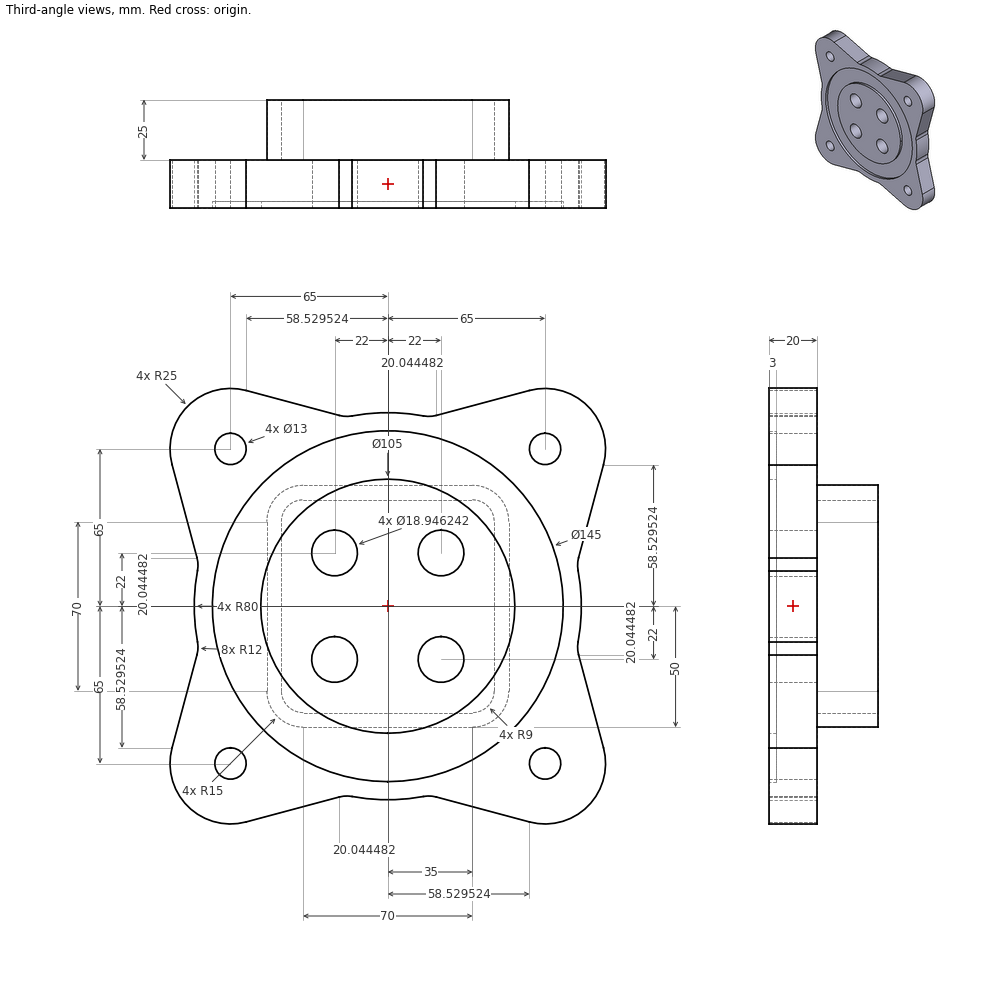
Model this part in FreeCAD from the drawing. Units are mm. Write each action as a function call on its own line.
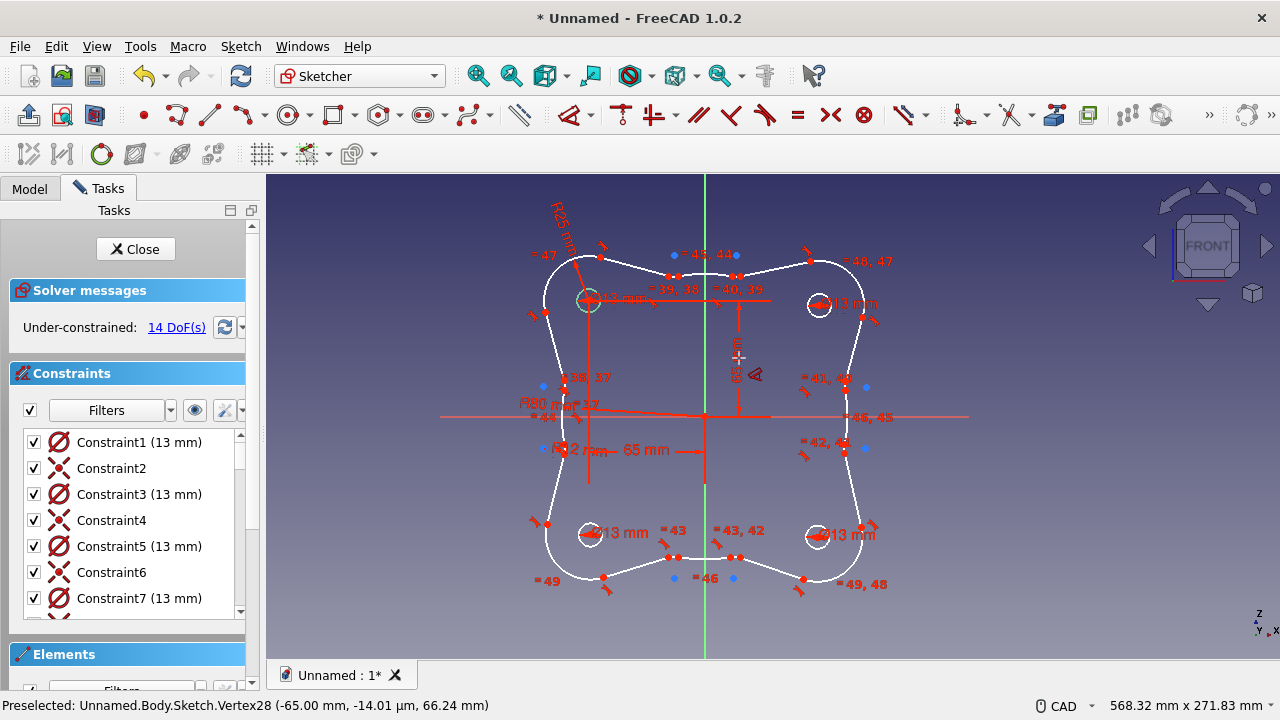
click(820, 306)
click(762, 451)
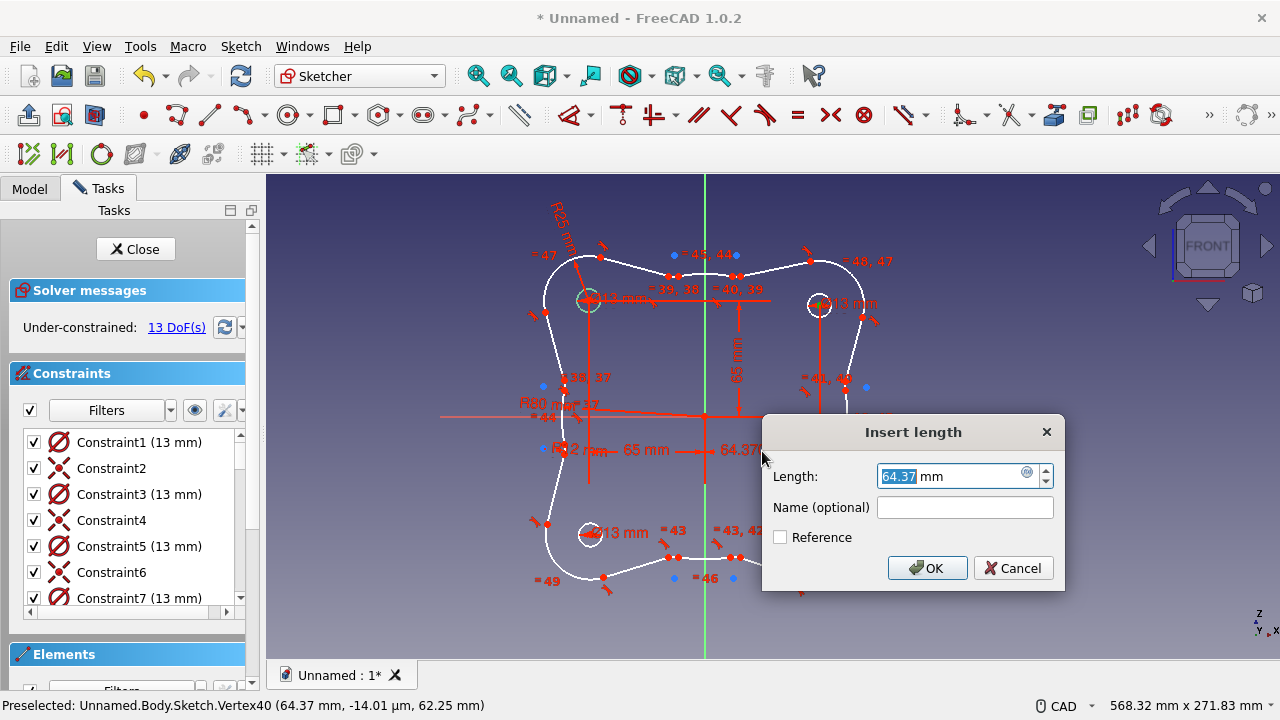
text(65)
key(Return)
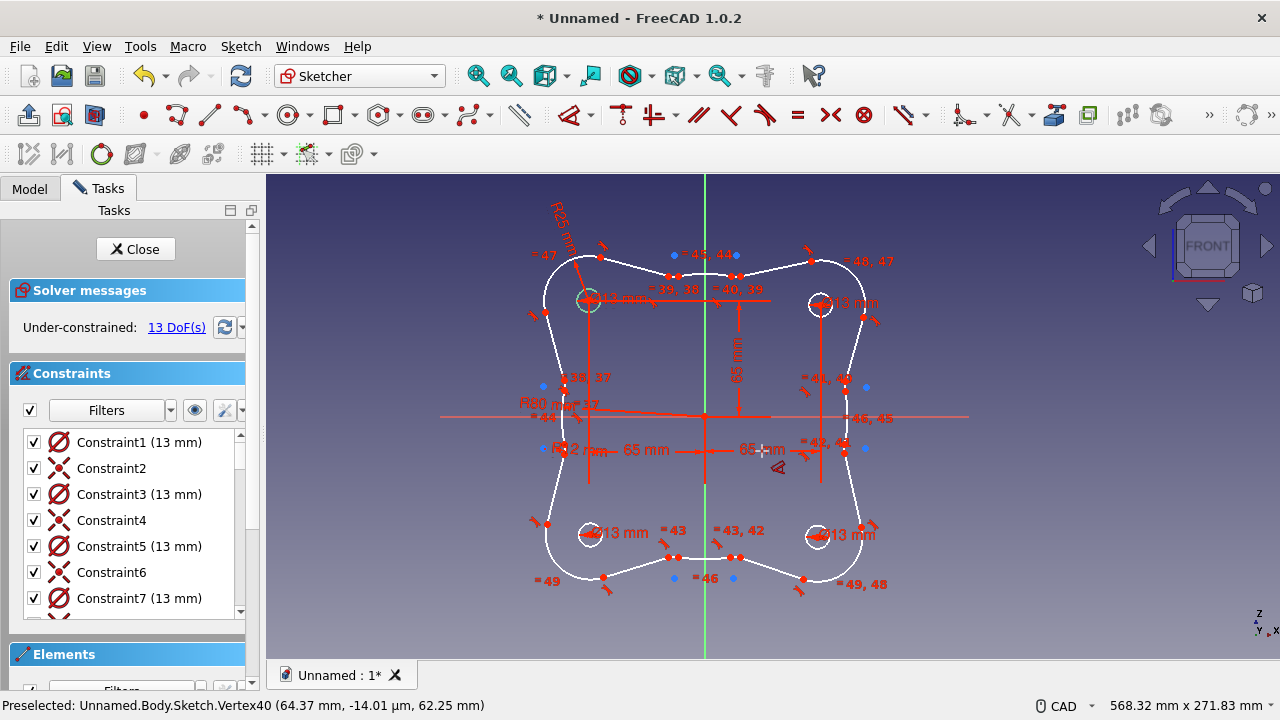
click(821, 305)
click(671, 335)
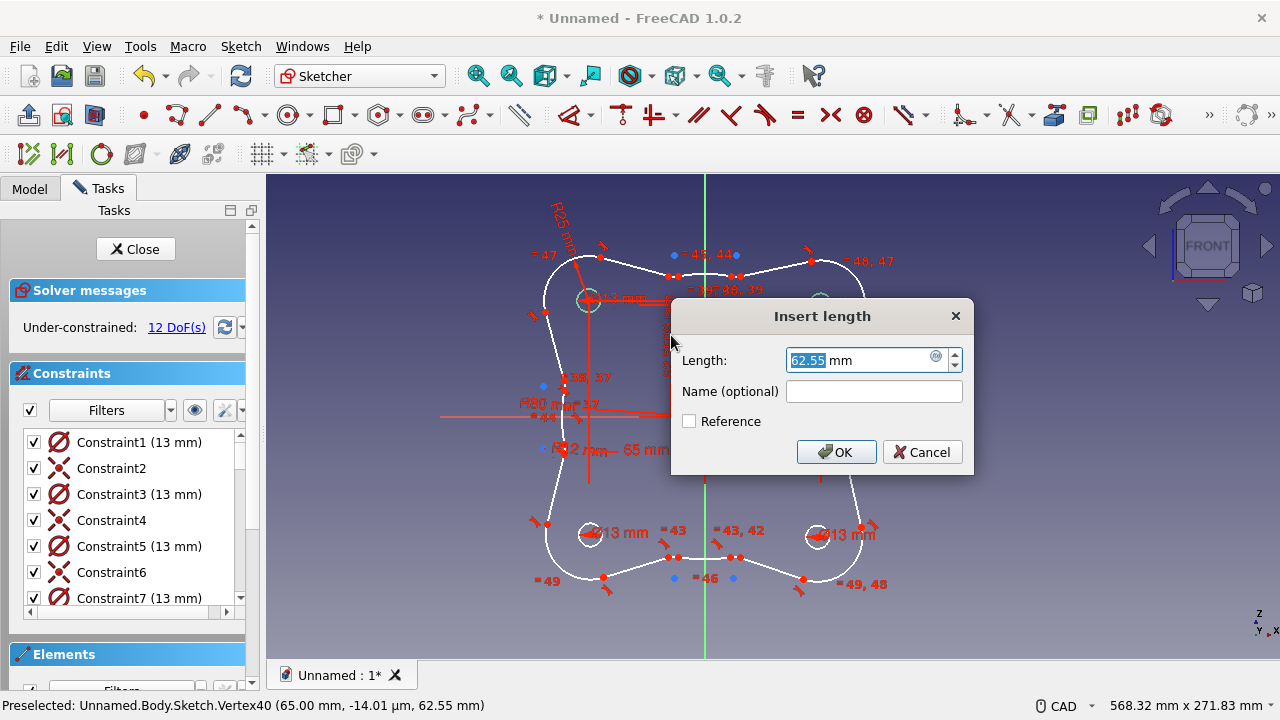
text(65)
key(Return)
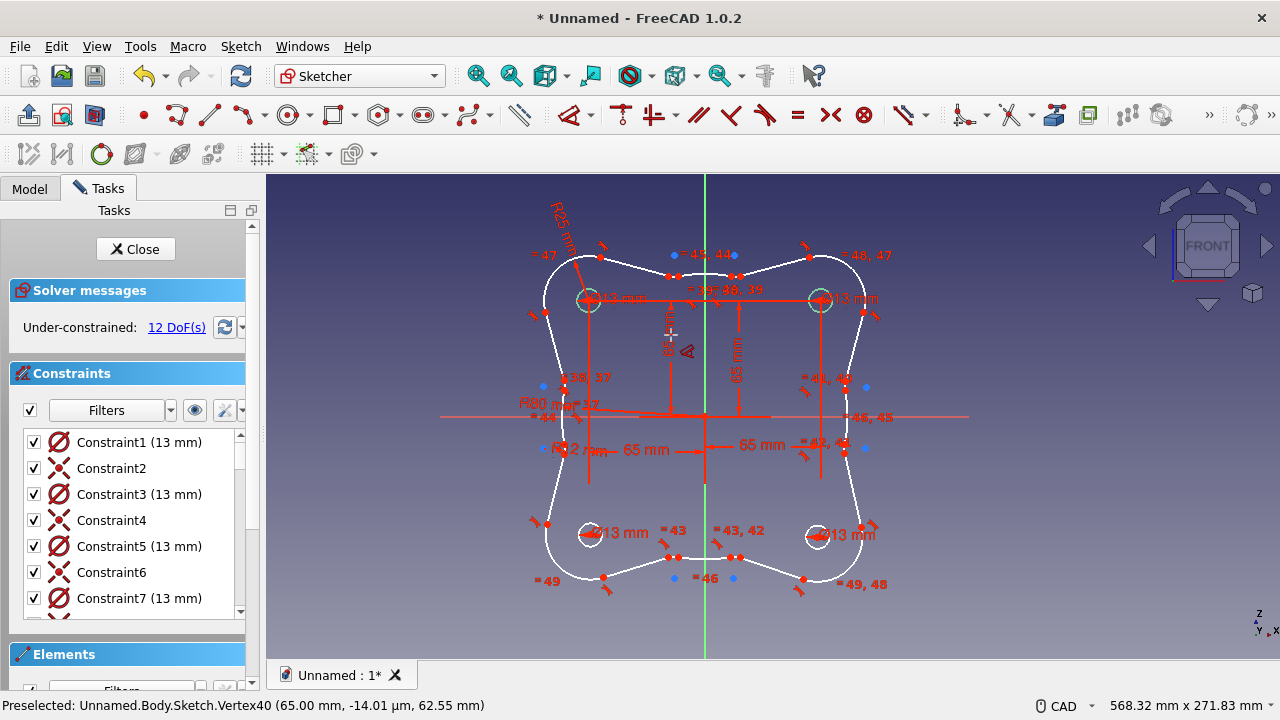
click(590, 535)
click(648, 383)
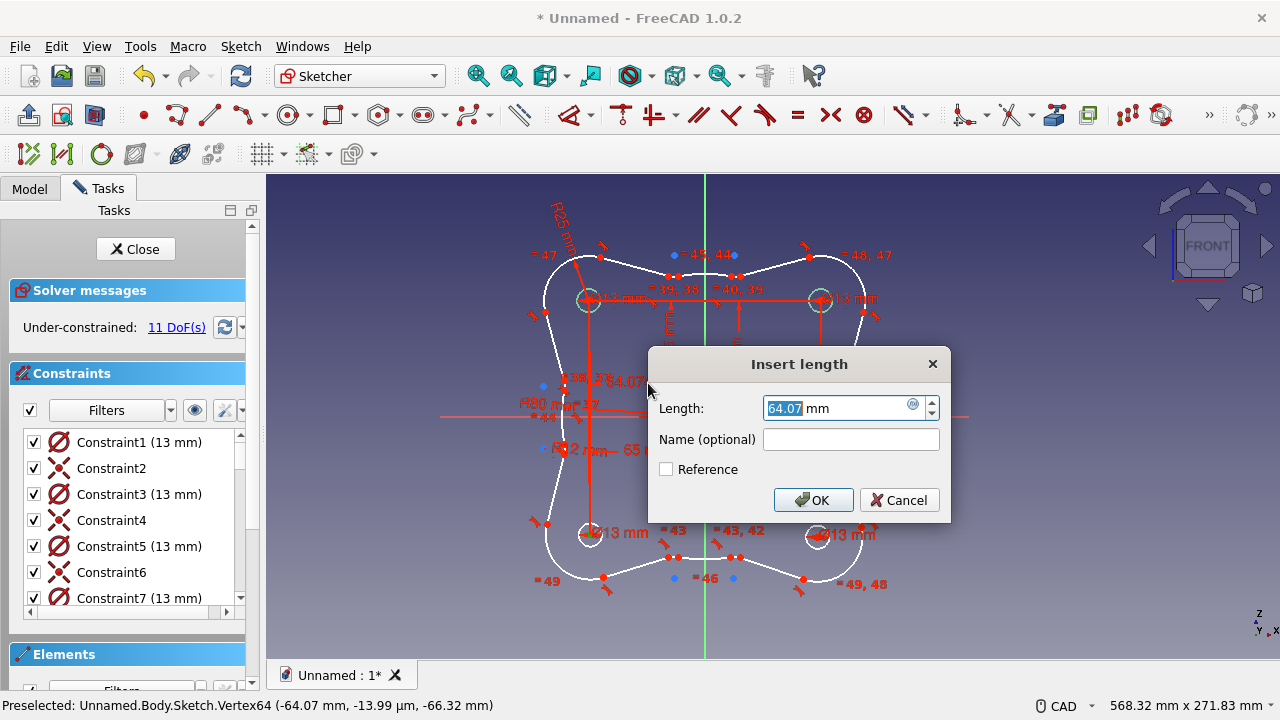
text(65)
key(Return)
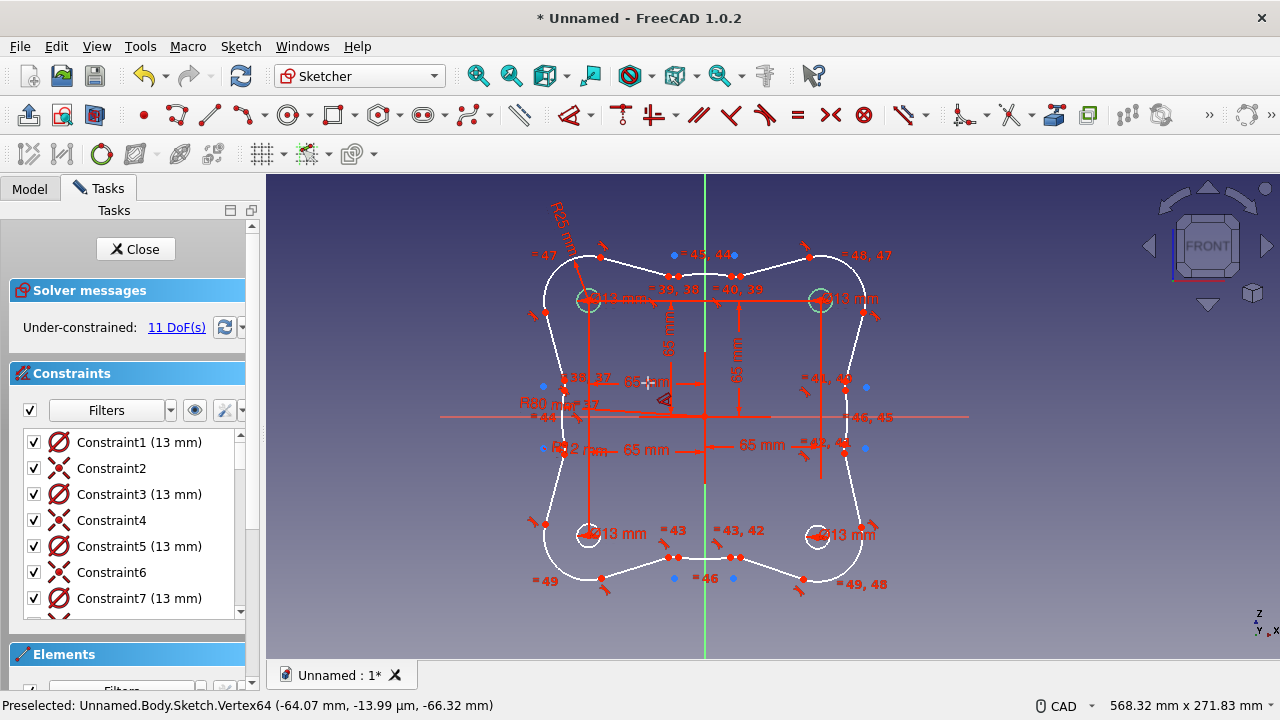
click(589, 536)
click(739, 476)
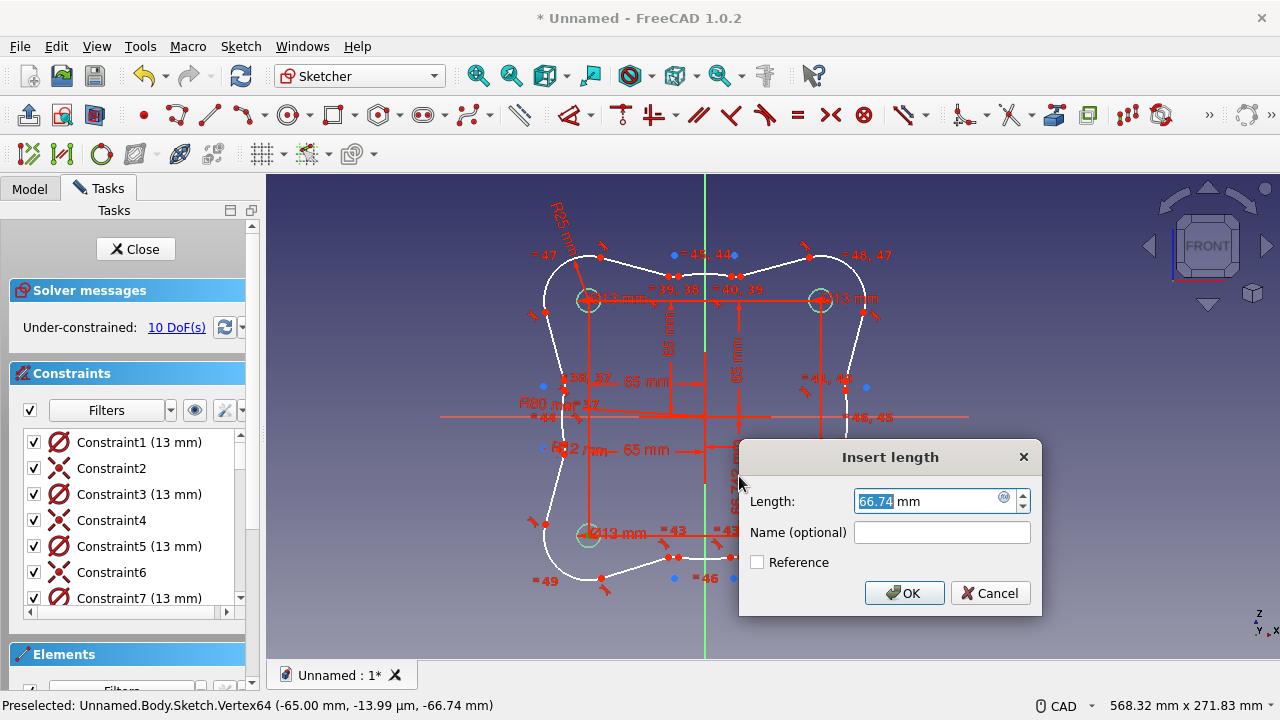
text(65)
key(Return)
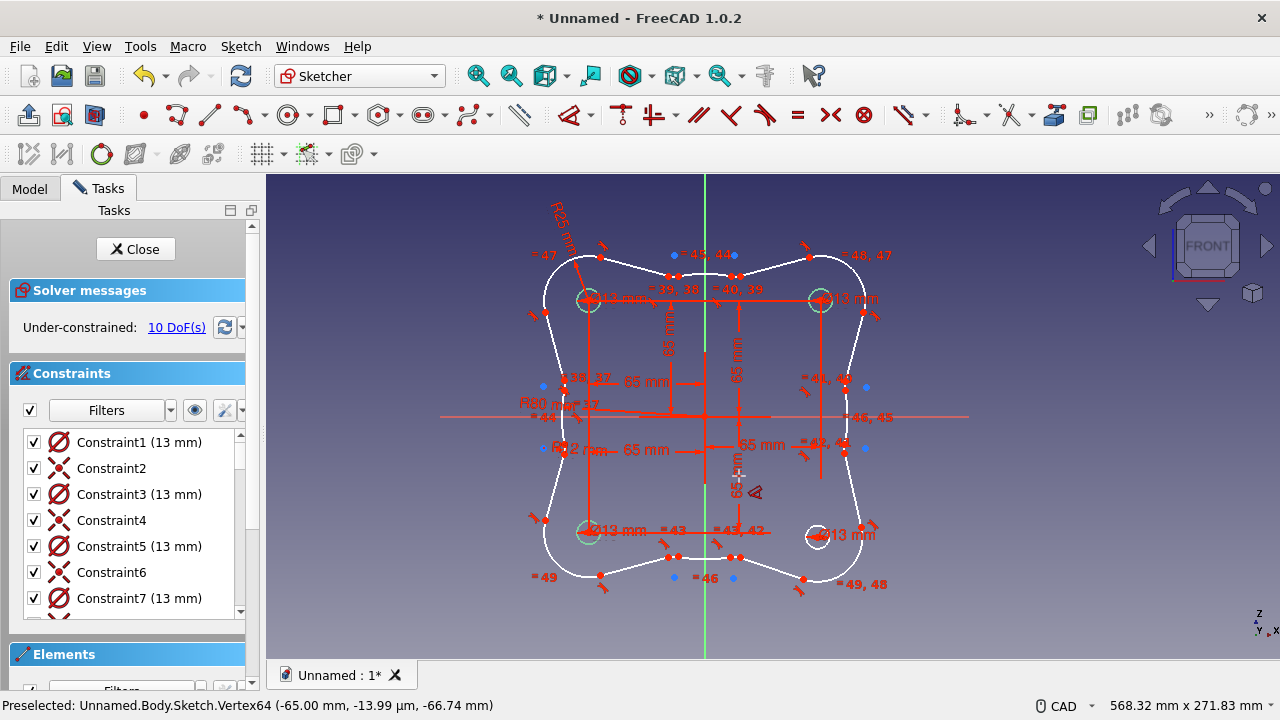
click(818, 537)
click(735, 571)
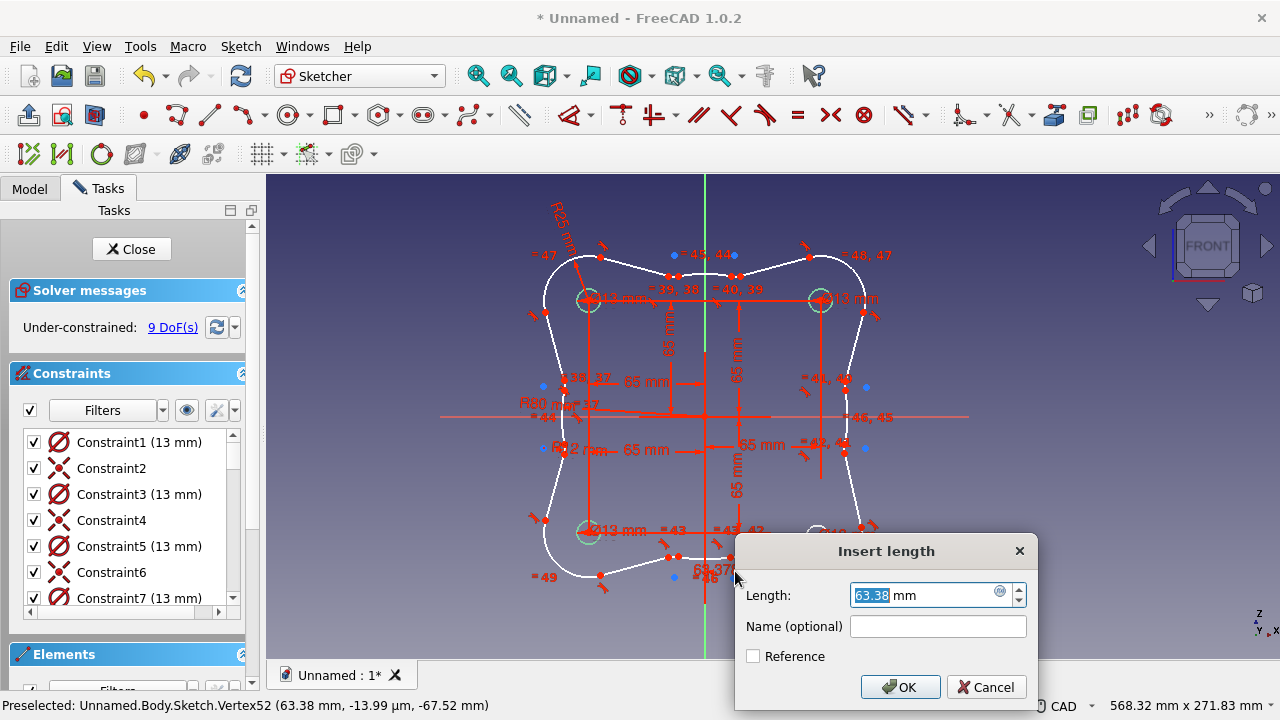
text(65)
key(Return)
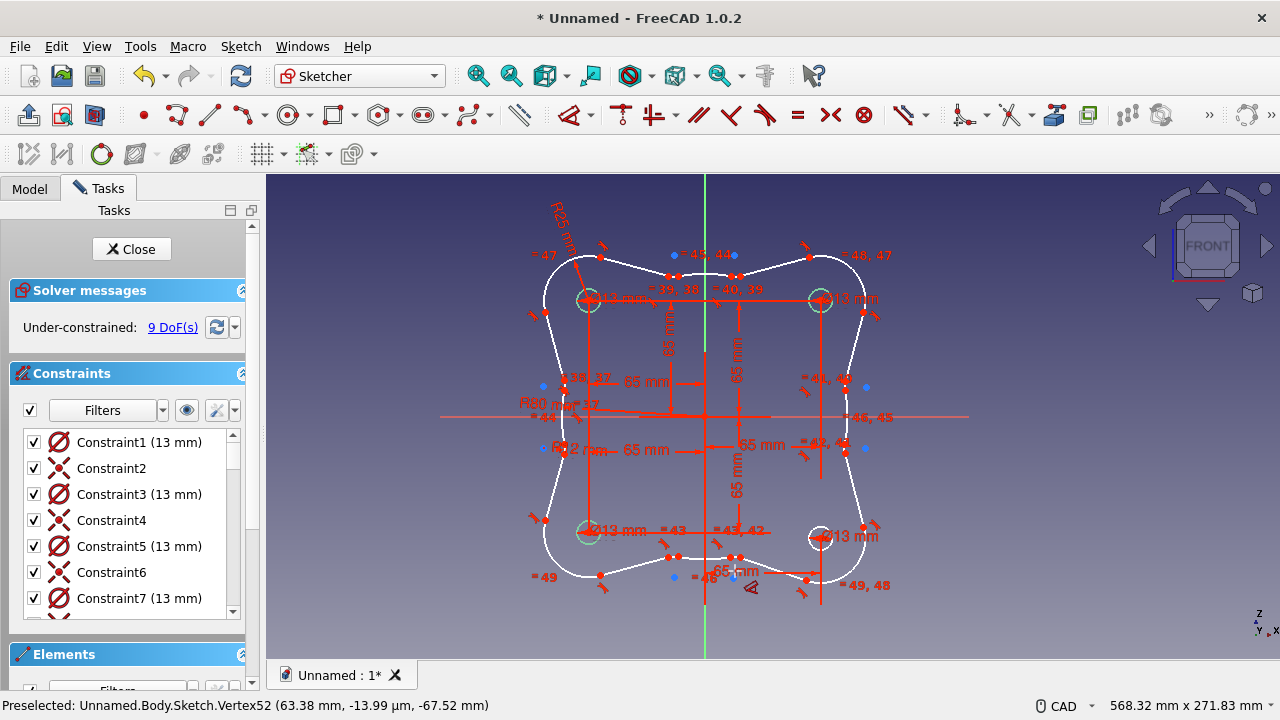
click(821, 538)
click(671, 506)